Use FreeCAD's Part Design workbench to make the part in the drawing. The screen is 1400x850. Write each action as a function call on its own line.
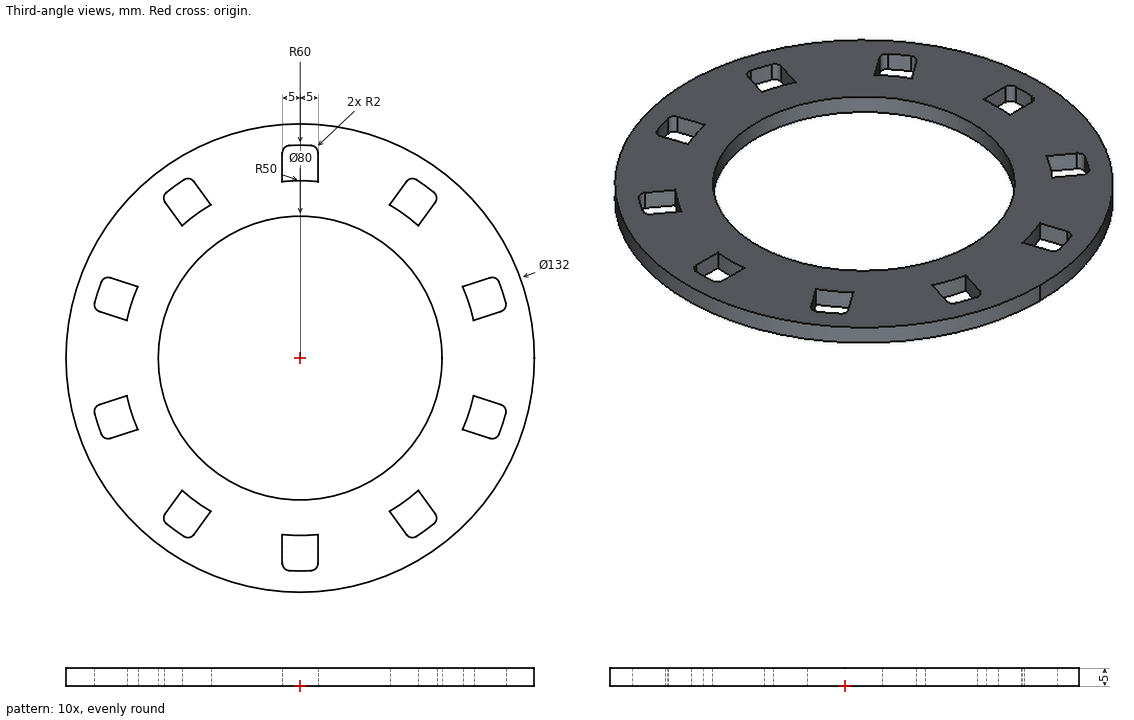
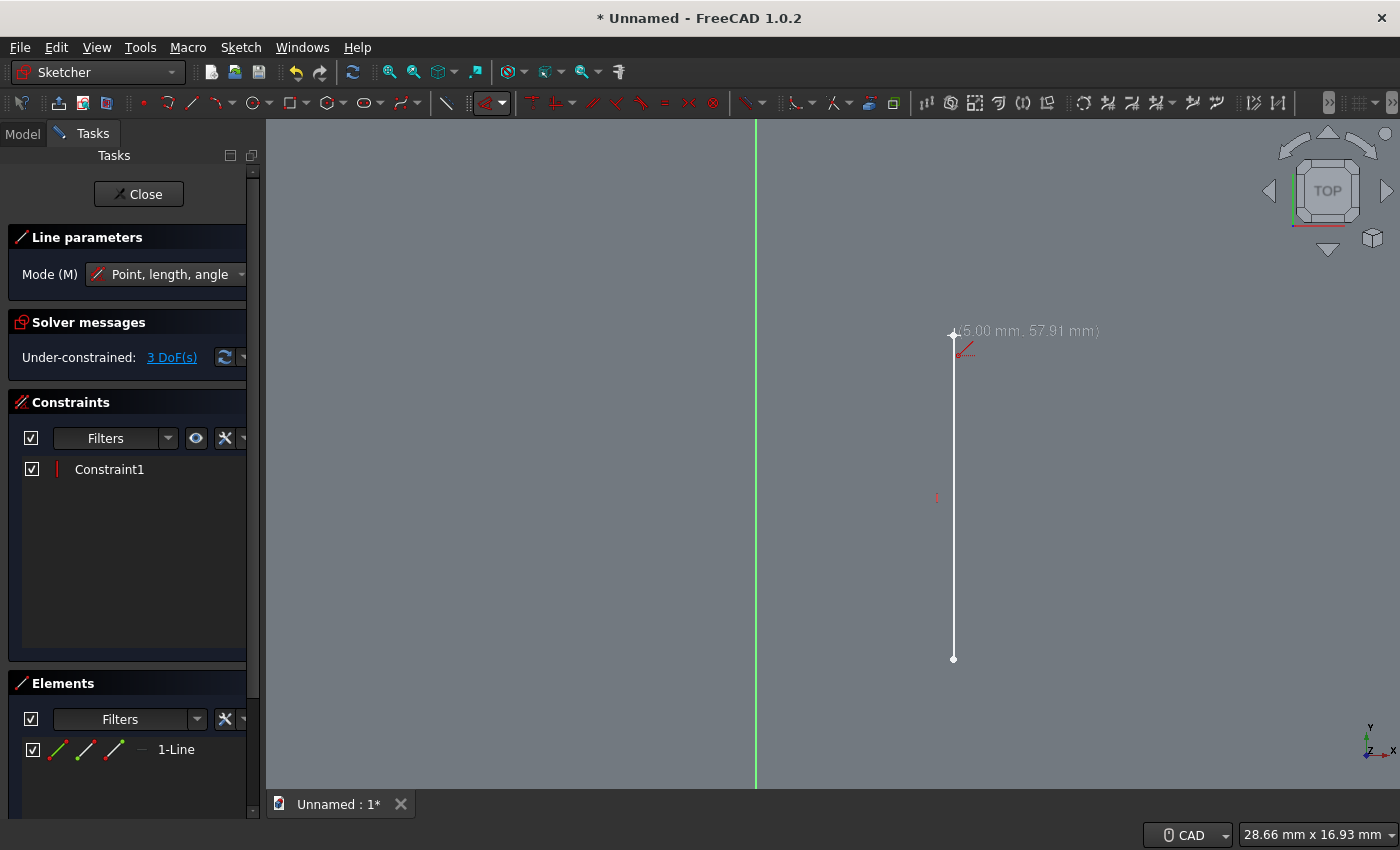
click(558, 335)
click(558, 659)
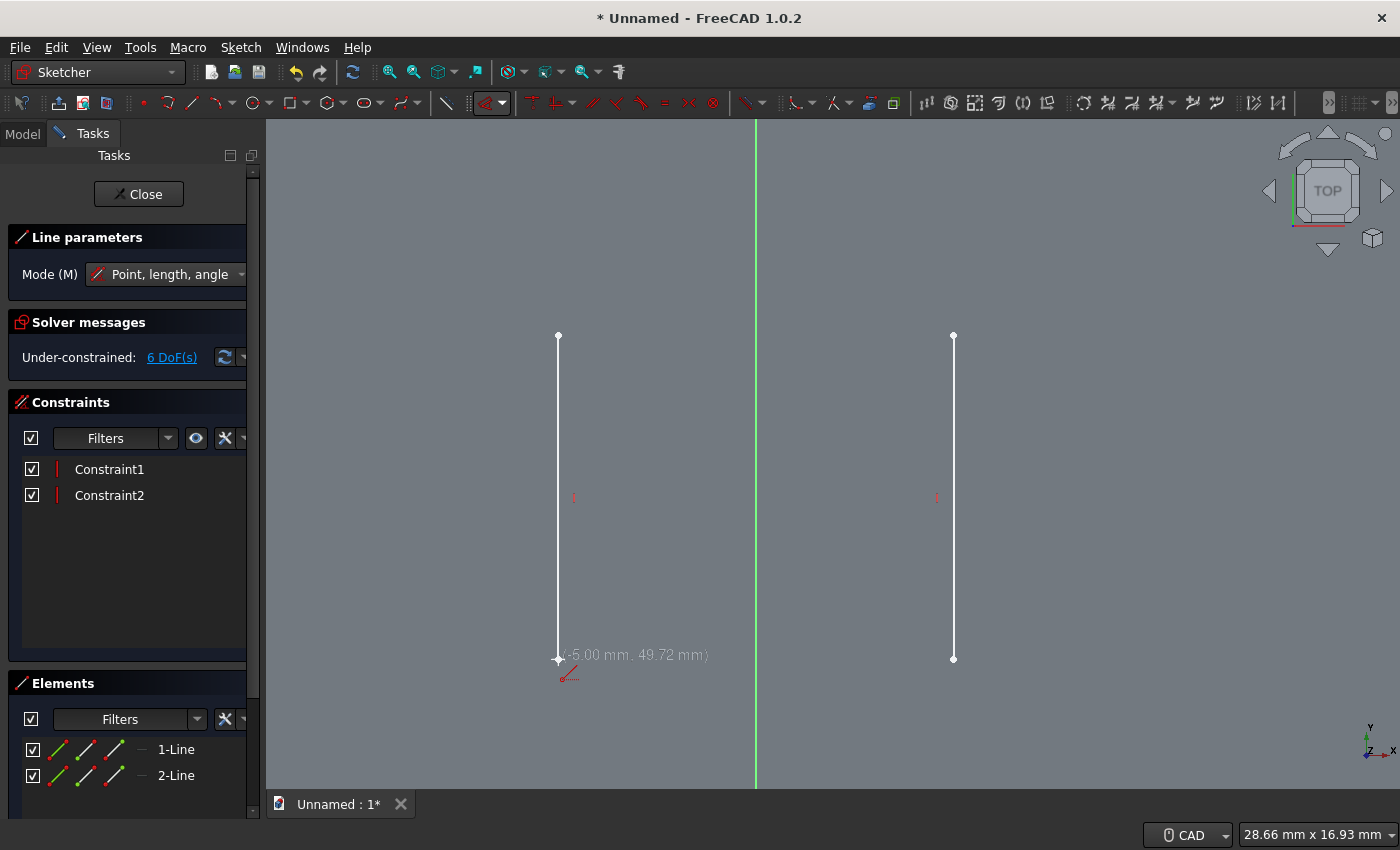
key(g)
key(3)
key(a)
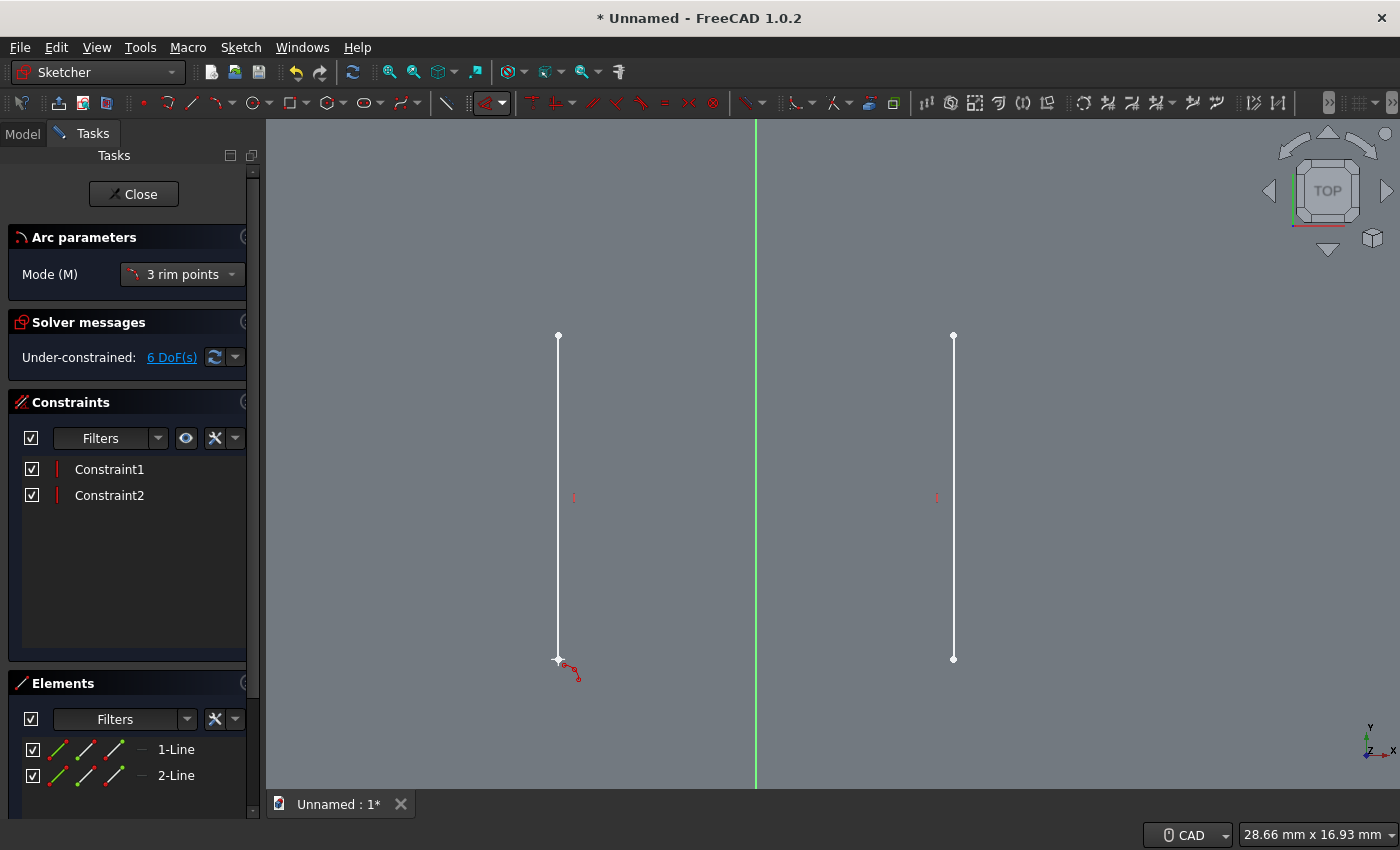
click(954, 336)
click(879, 256)
click(932, 281)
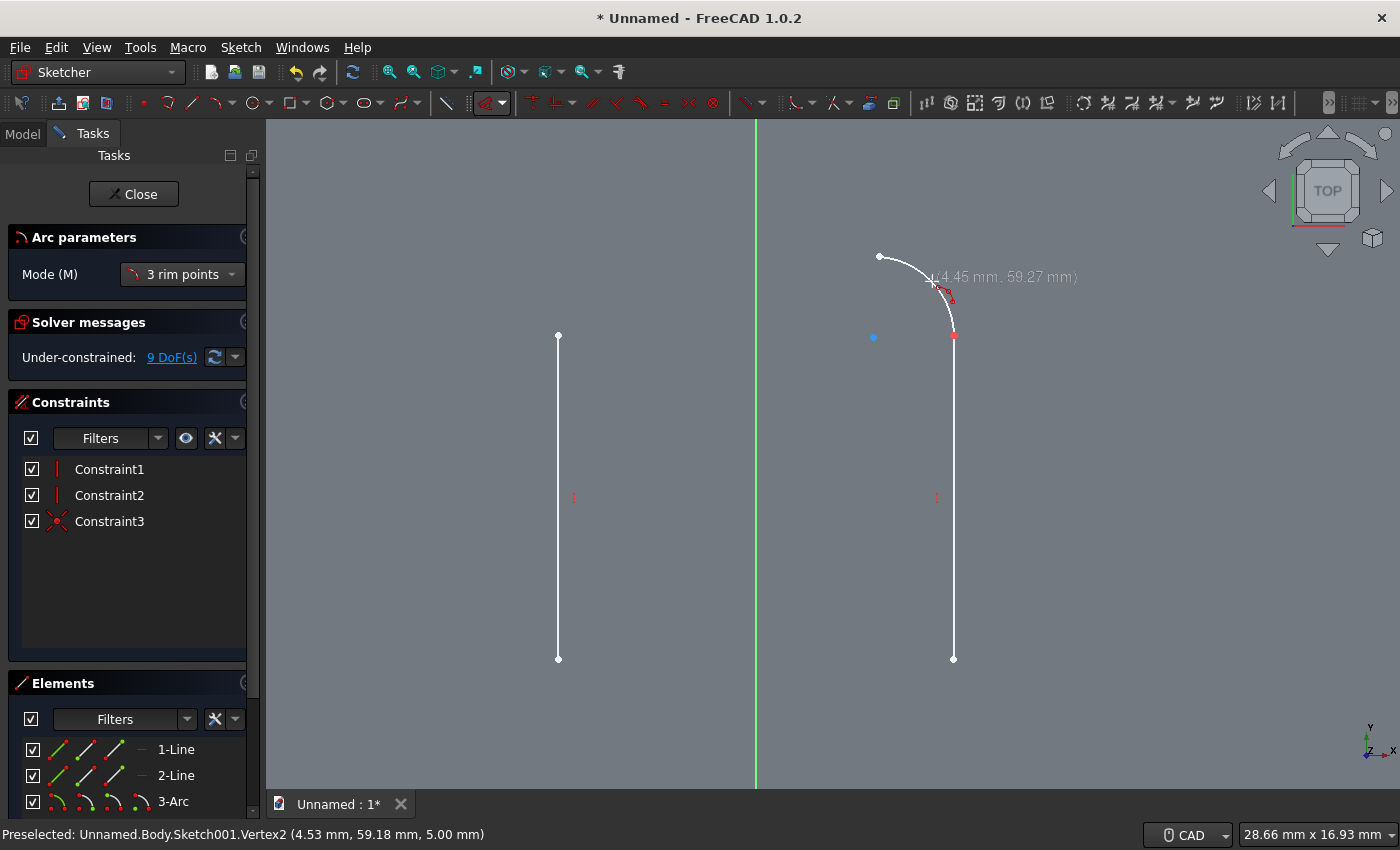
click(879, 257)
click(633, 256)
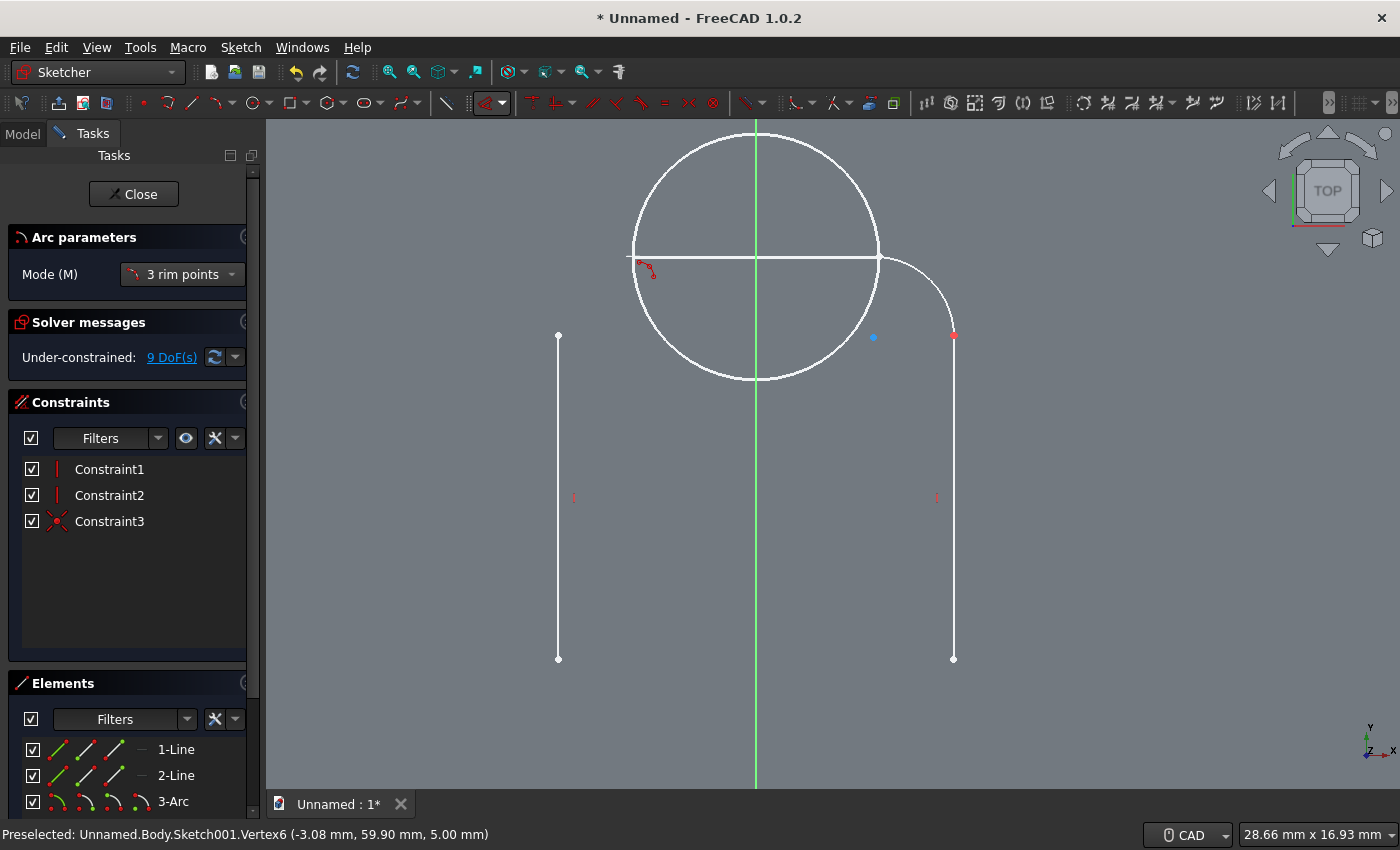
scroll(781, 253, up, 9)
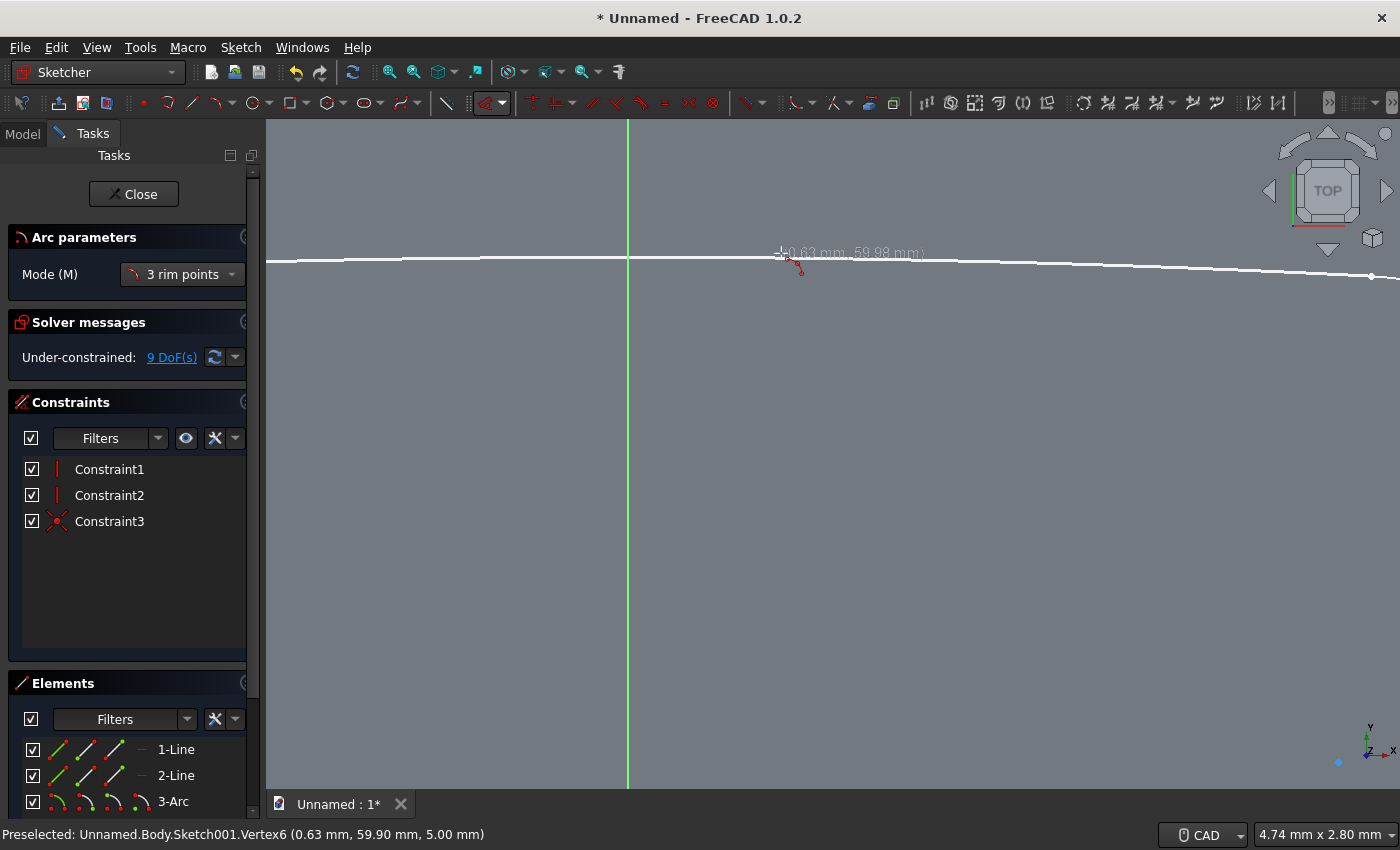
click(776, 254)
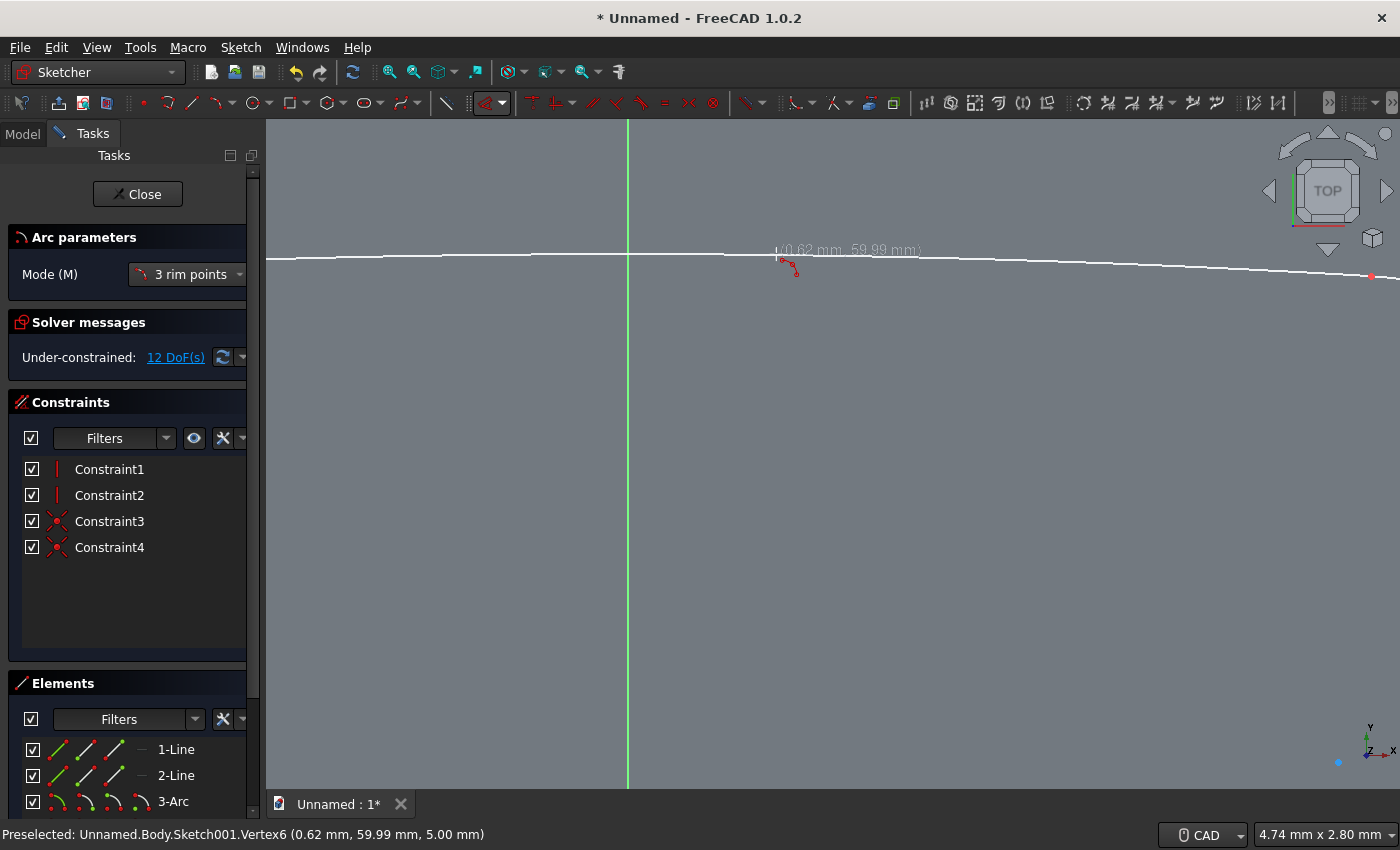
scroll(792, 251, down, 9)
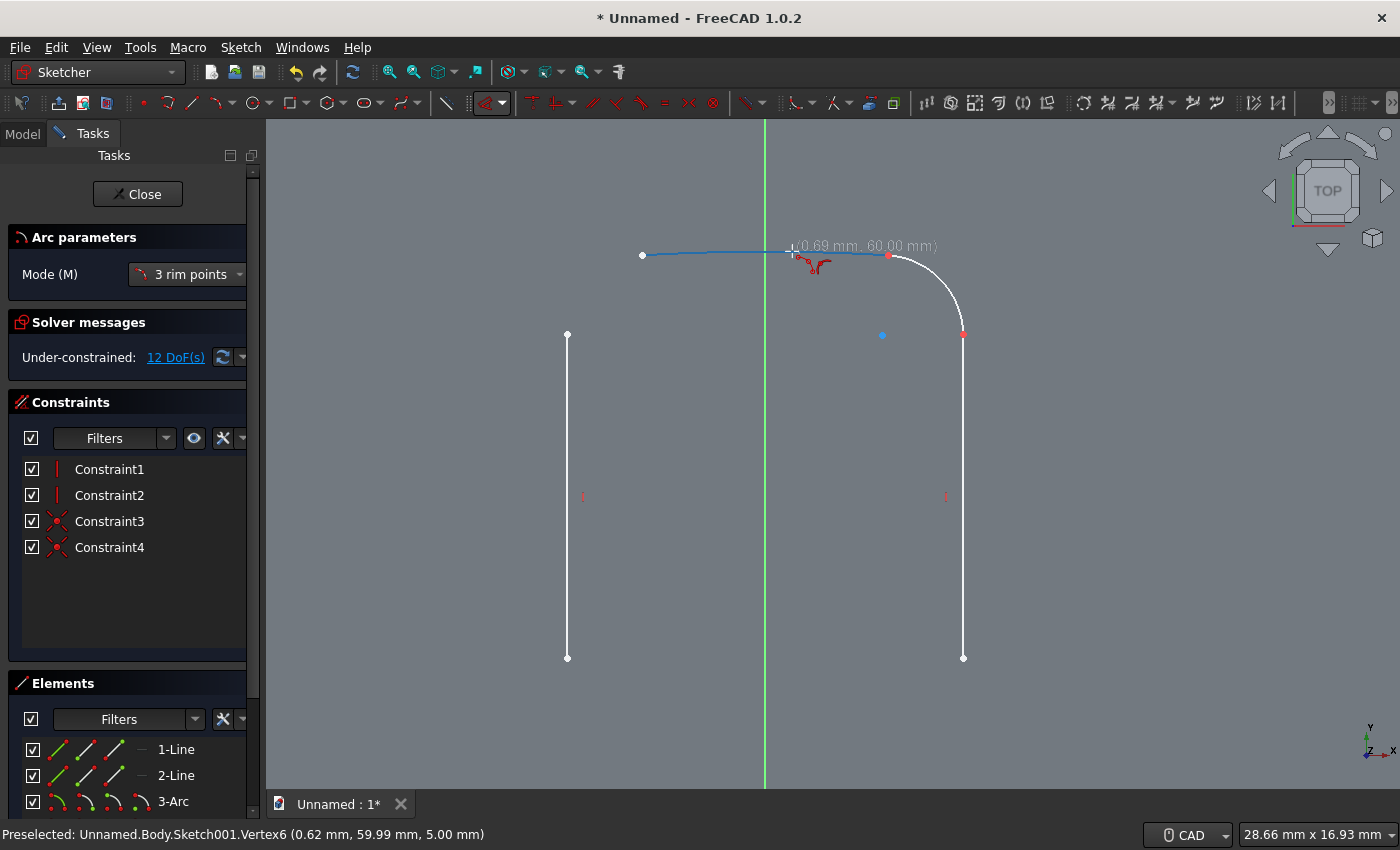
click(642, 255)
click(567, 334)
click(589, 279)